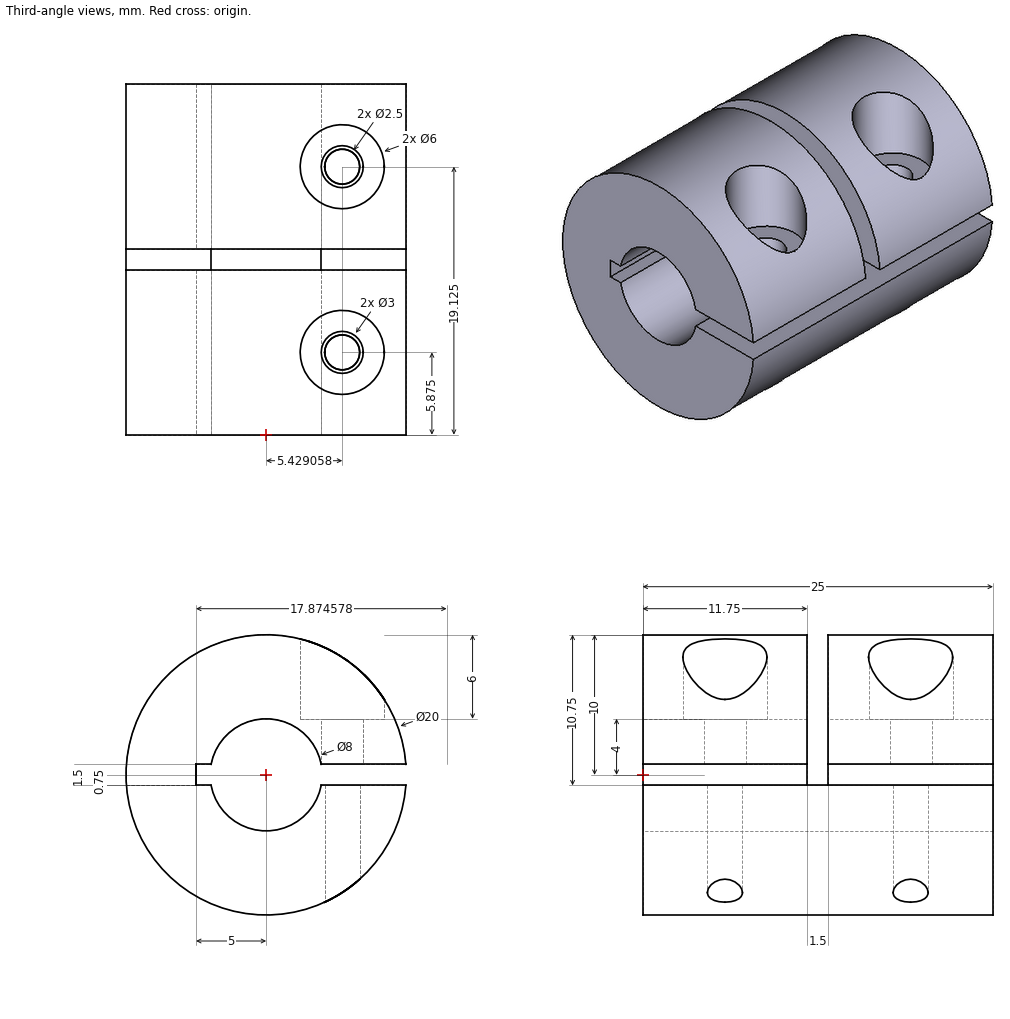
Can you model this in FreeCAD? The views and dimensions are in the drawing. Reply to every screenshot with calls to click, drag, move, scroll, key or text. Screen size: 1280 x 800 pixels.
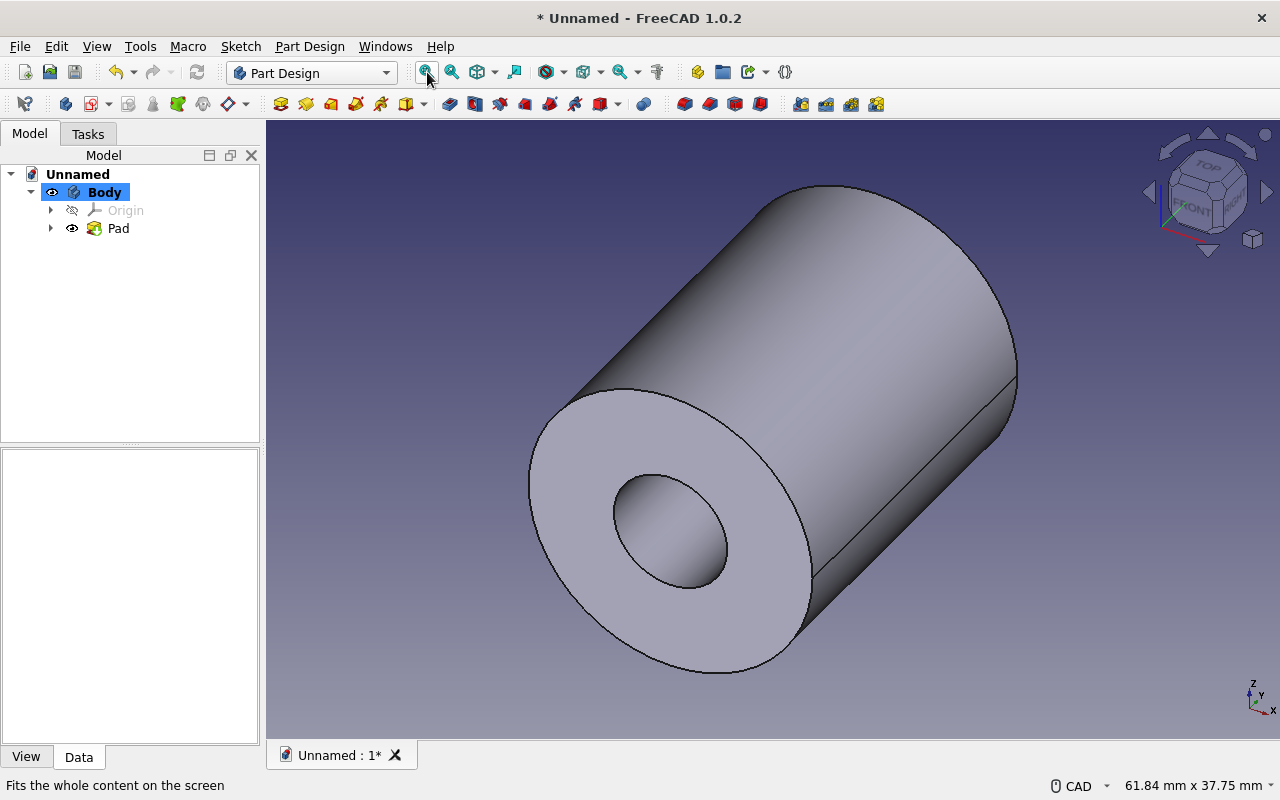
click(90, 104)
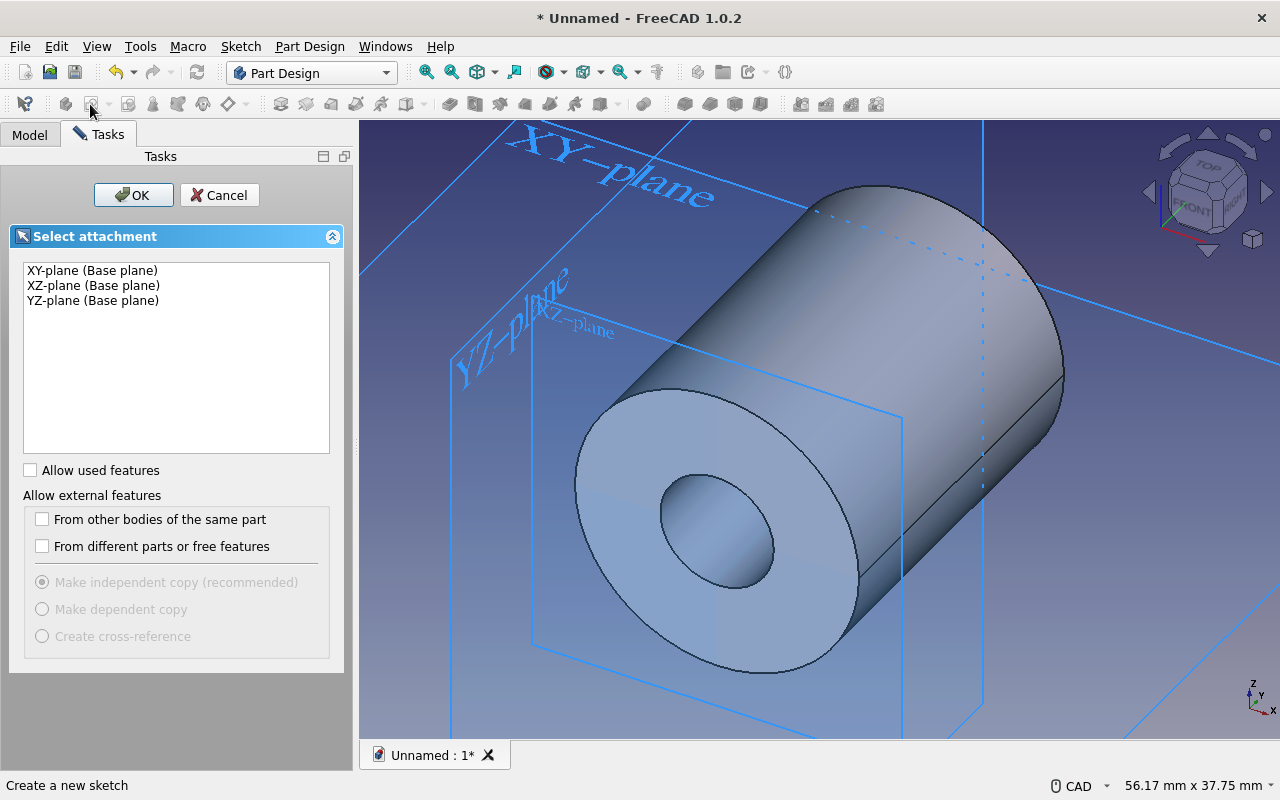
click(84, 300)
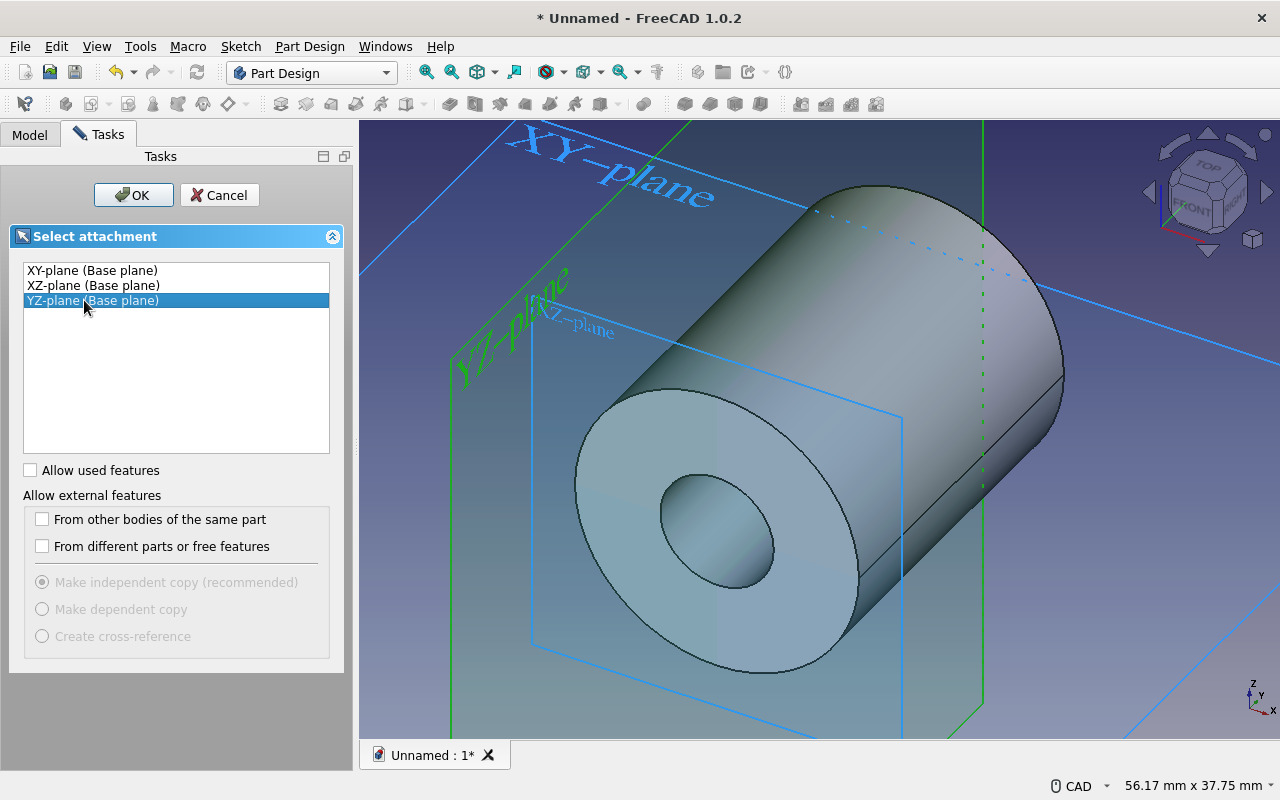
click(134, 195)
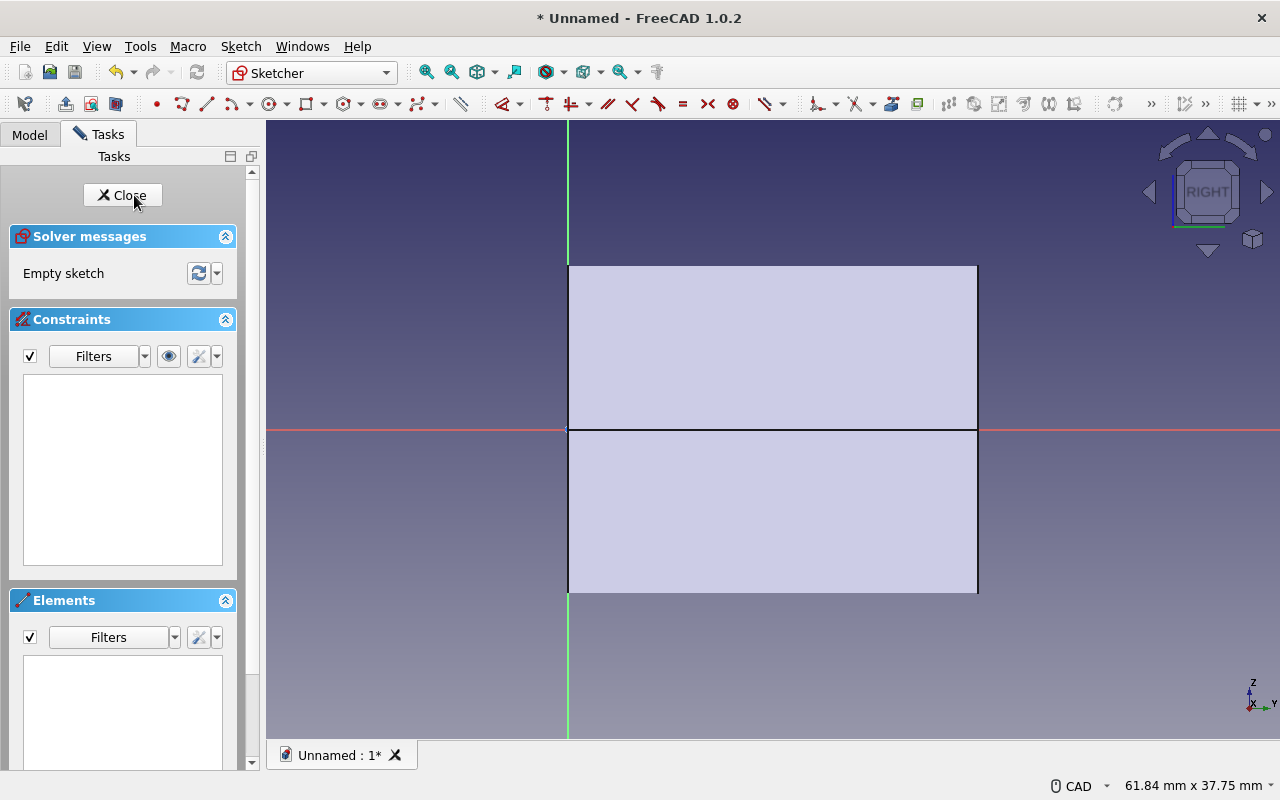
click(116, 104)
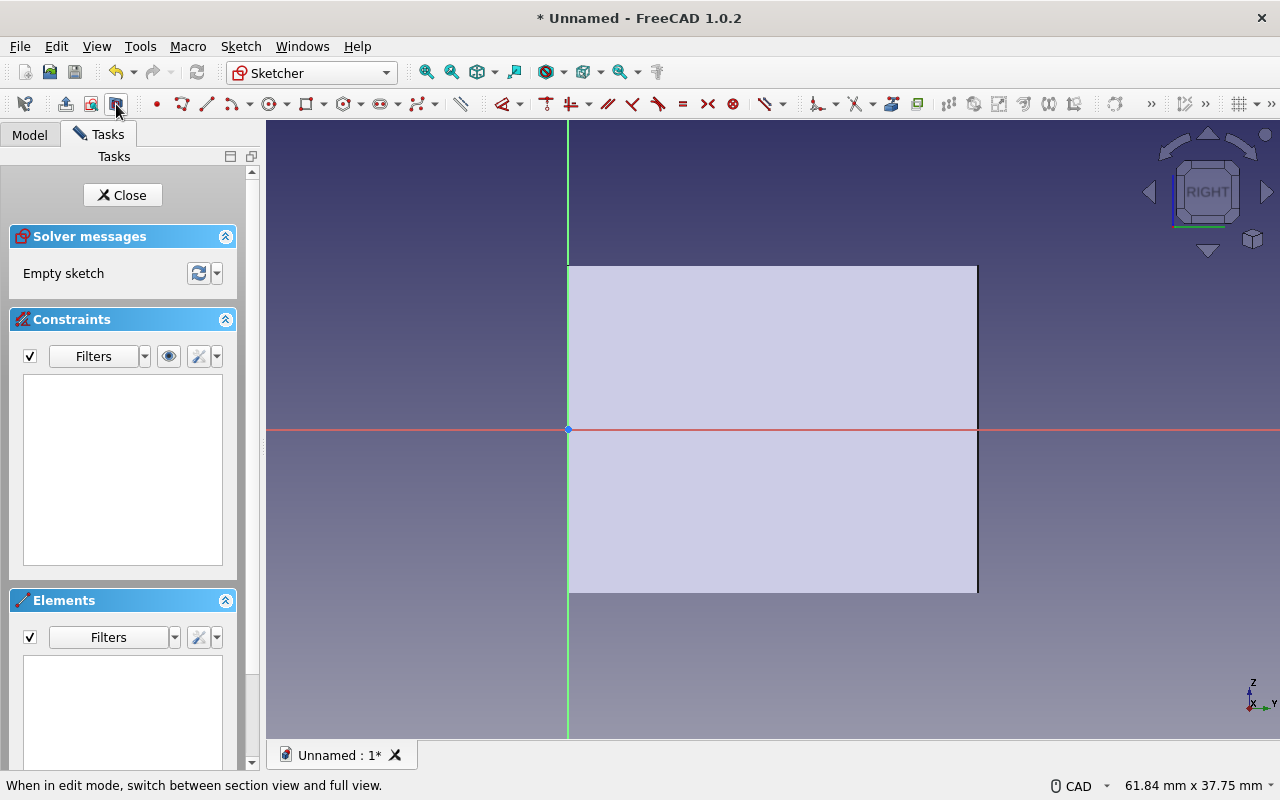
scroll(654, 292, up, 4)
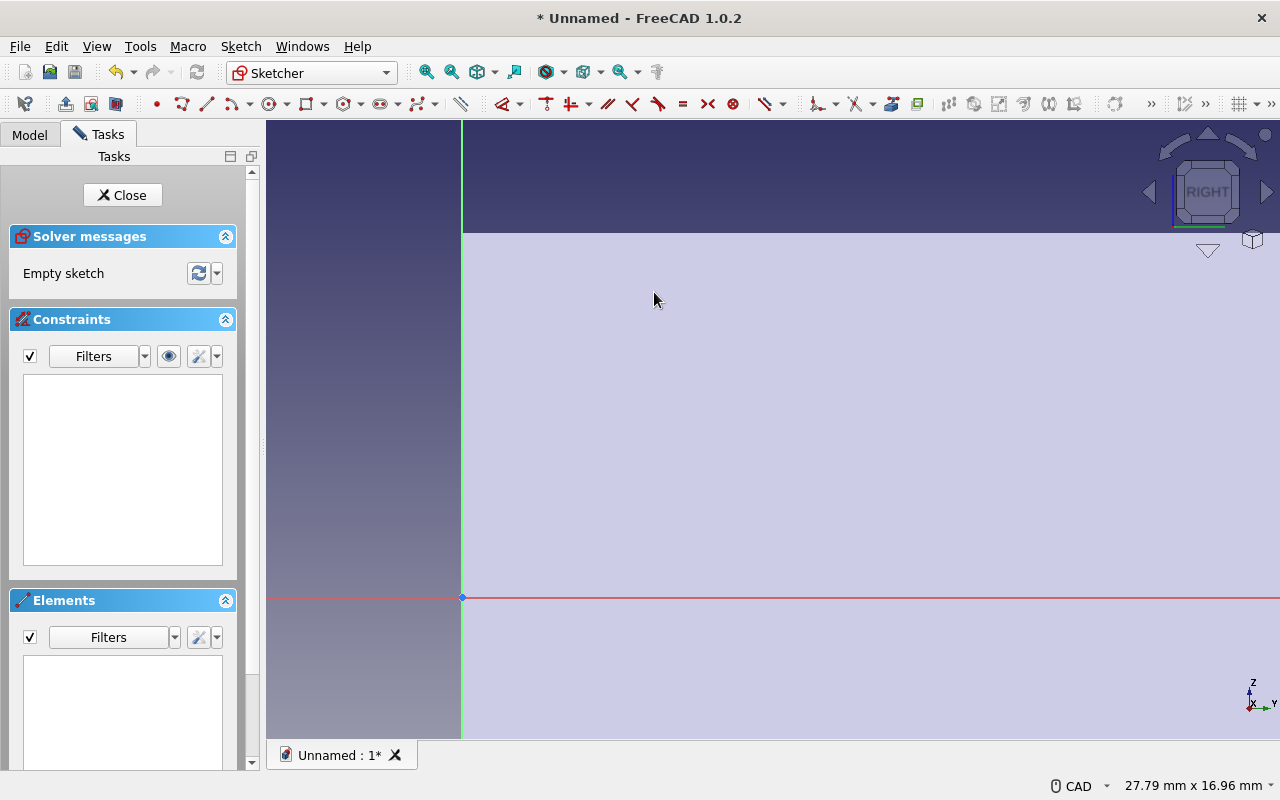
click(306, 104)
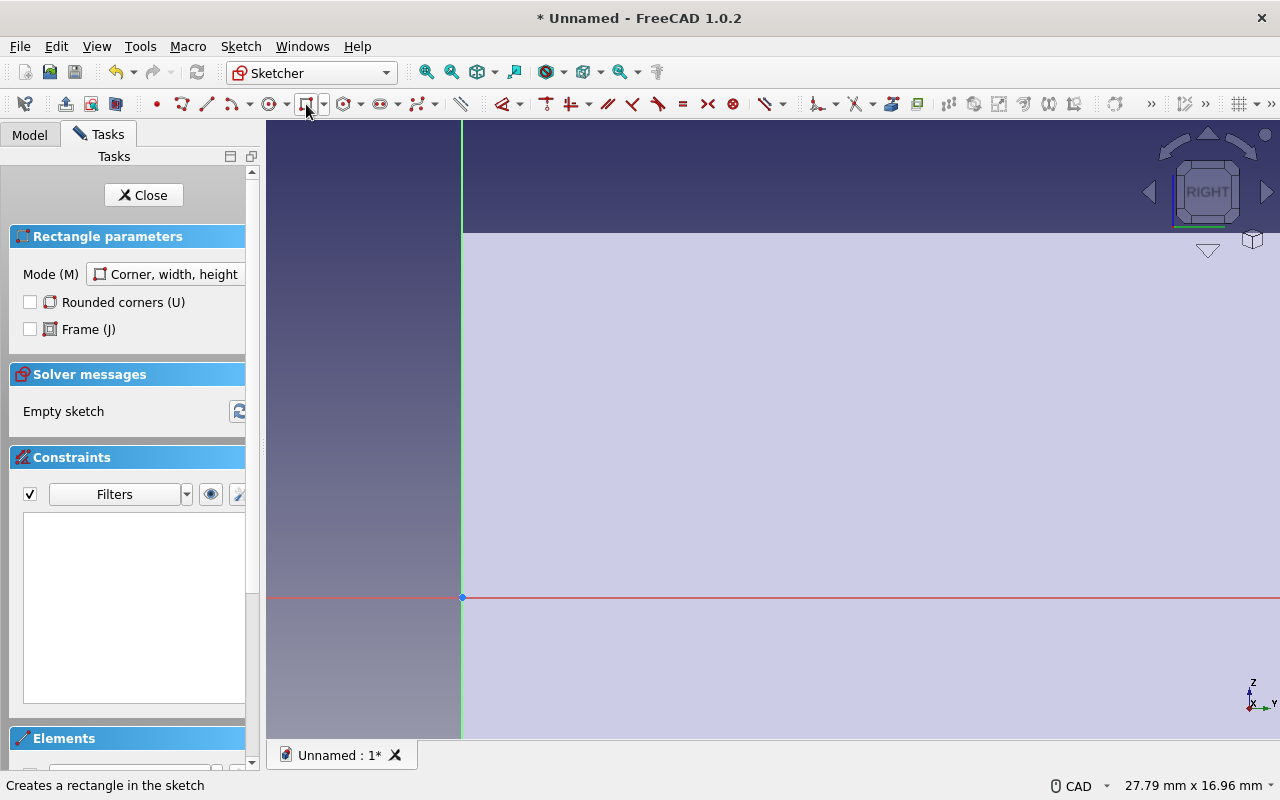
click(891, 233)
click(946, 625)
key(Escape)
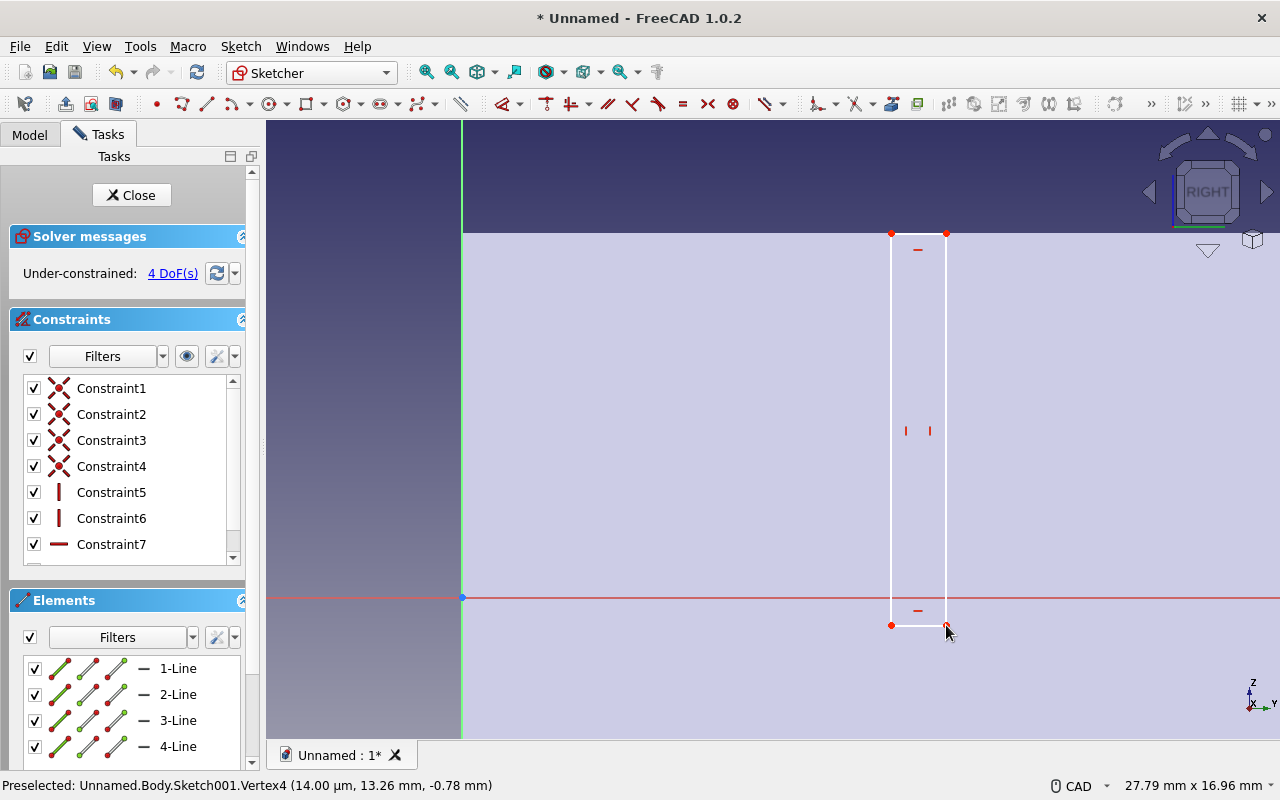
click(907, 626)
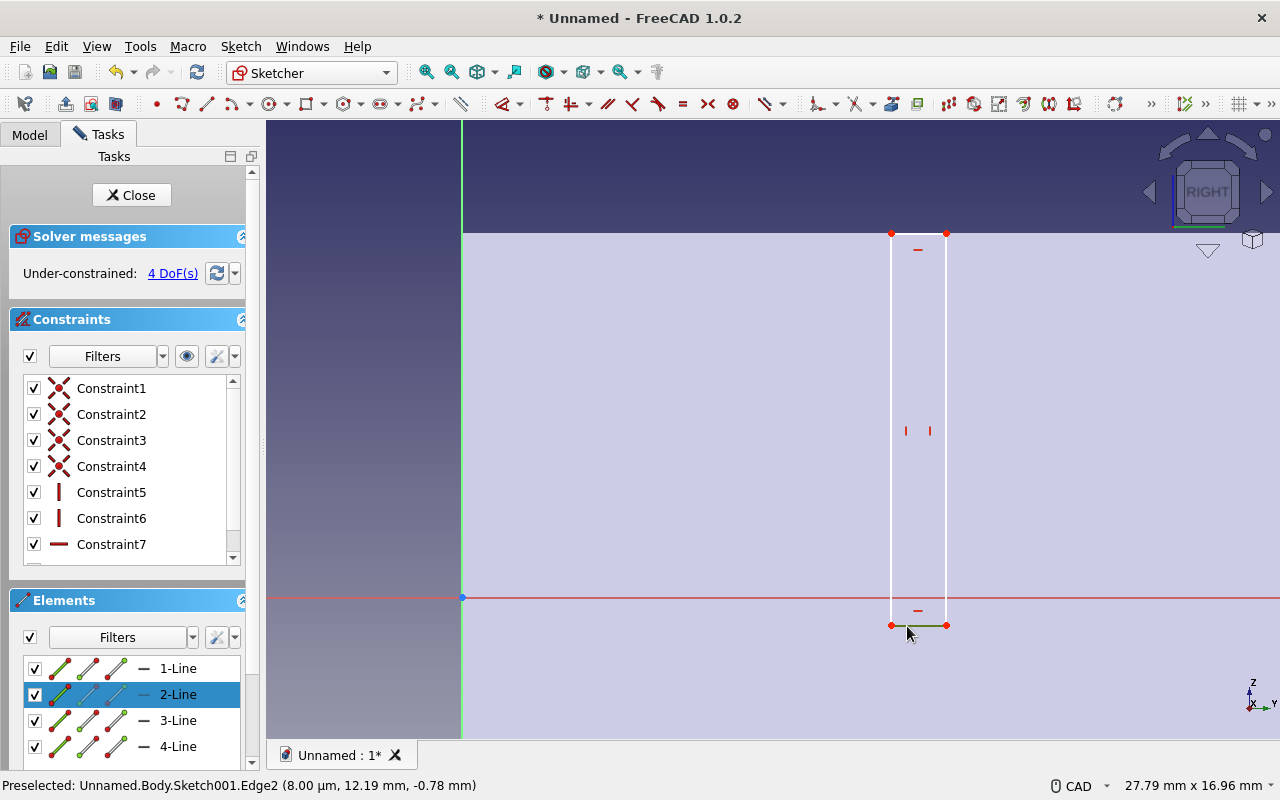
key(l)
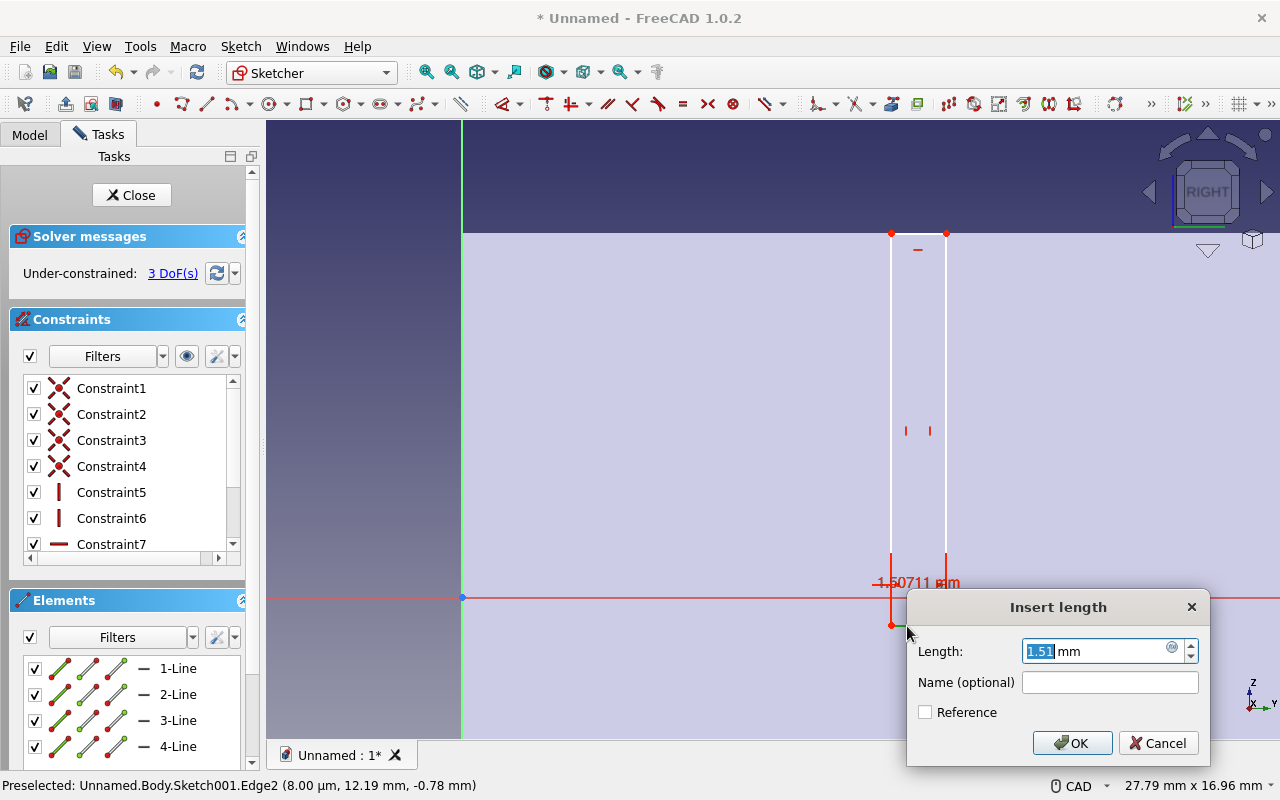
text(1.5)
key(Return)